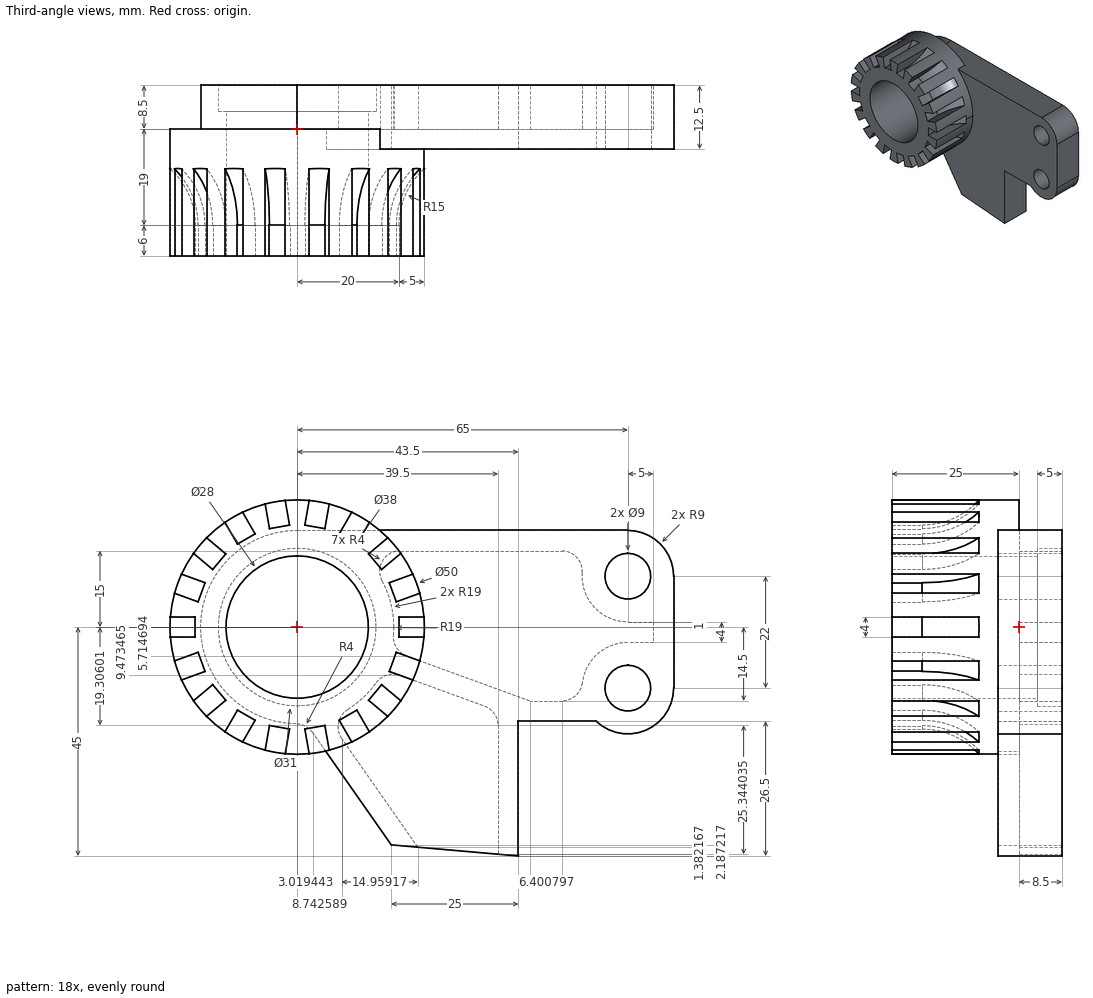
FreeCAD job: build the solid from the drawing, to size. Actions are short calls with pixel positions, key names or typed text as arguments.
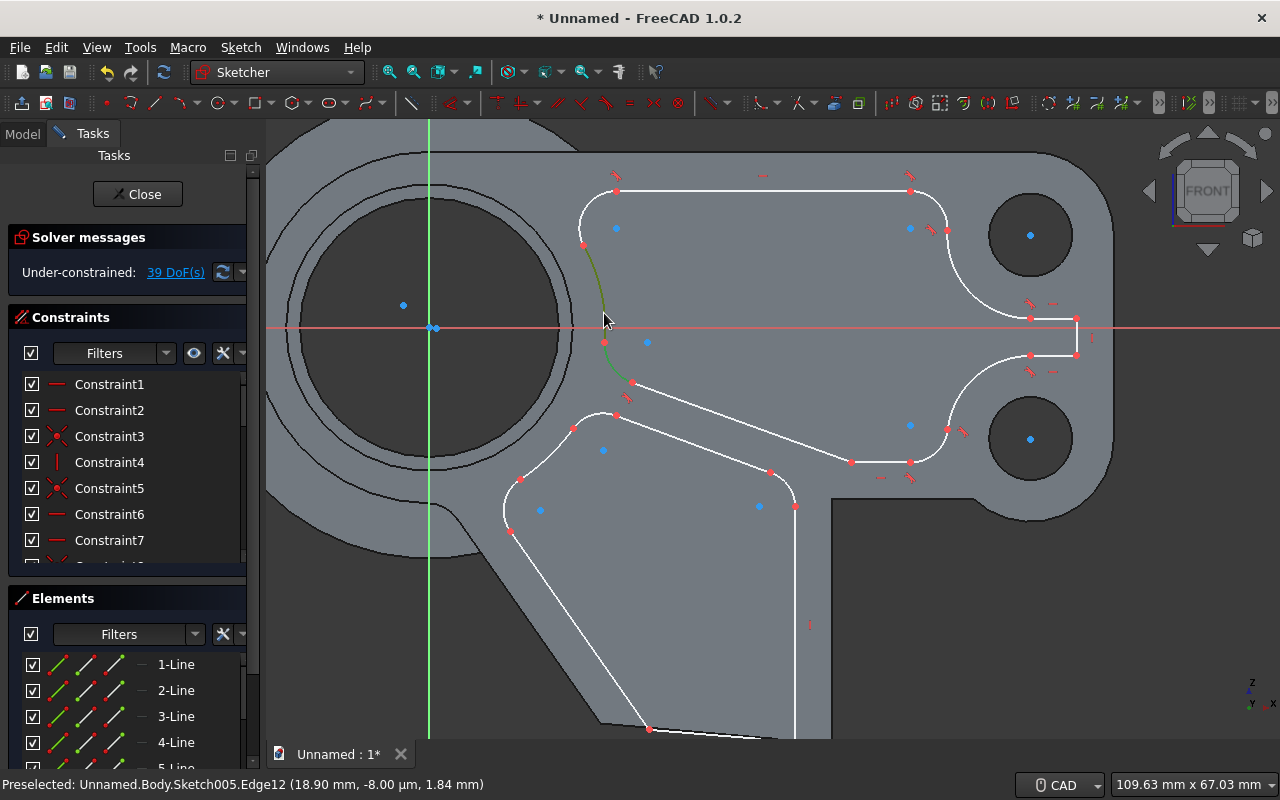
click(606, 104)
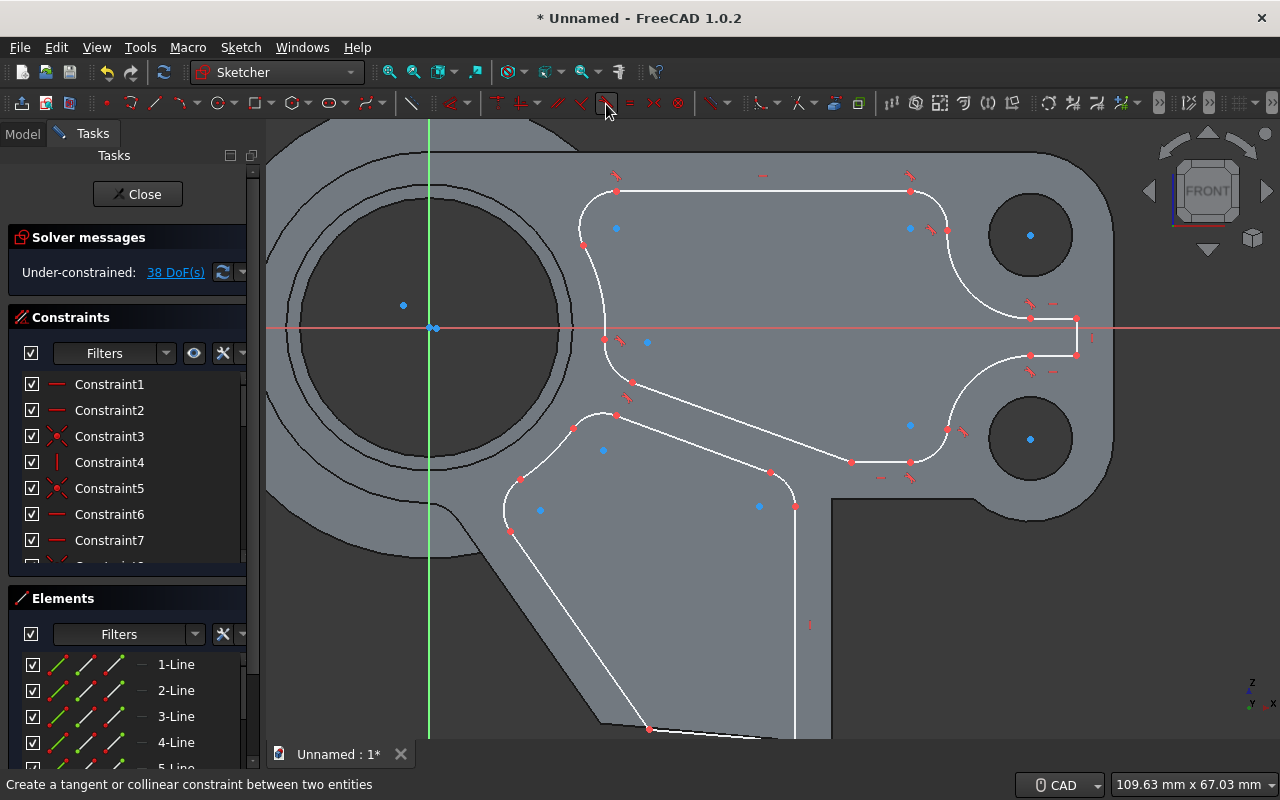
click(604, 310)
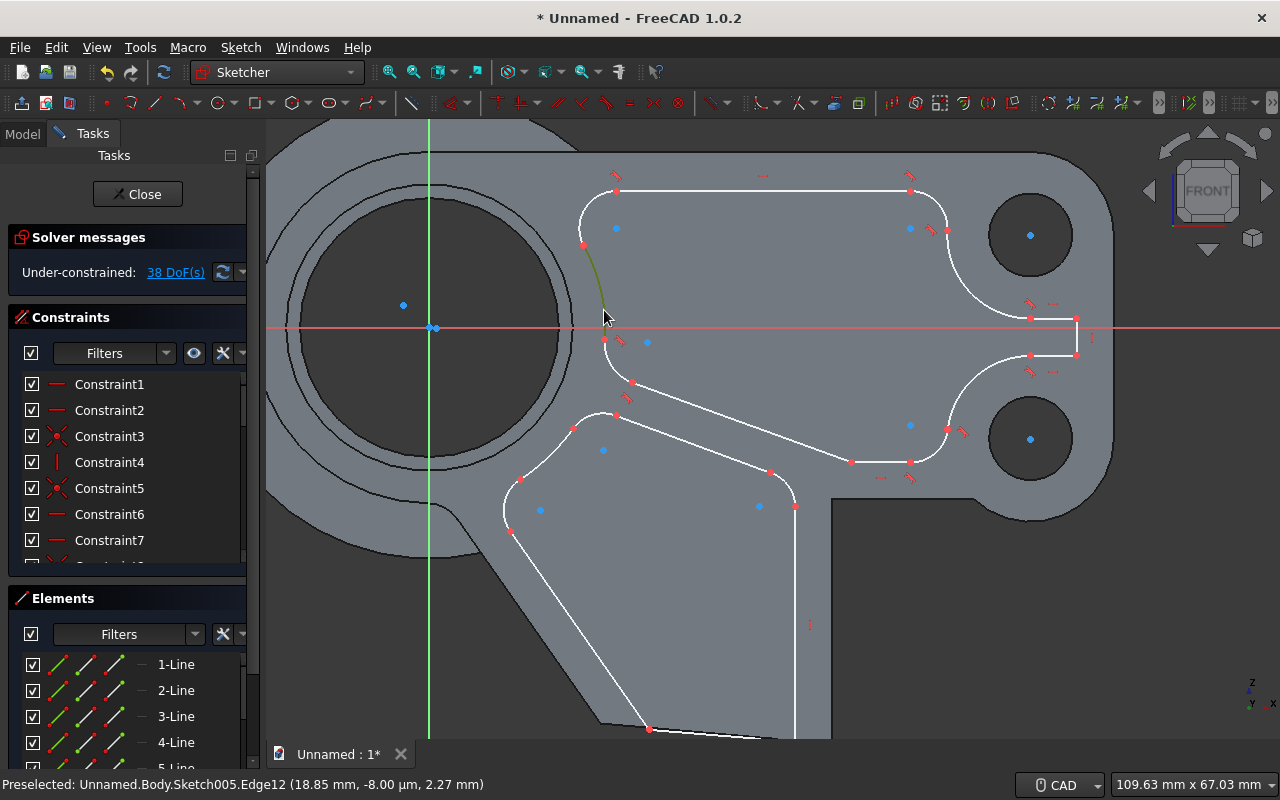
click(595, 198)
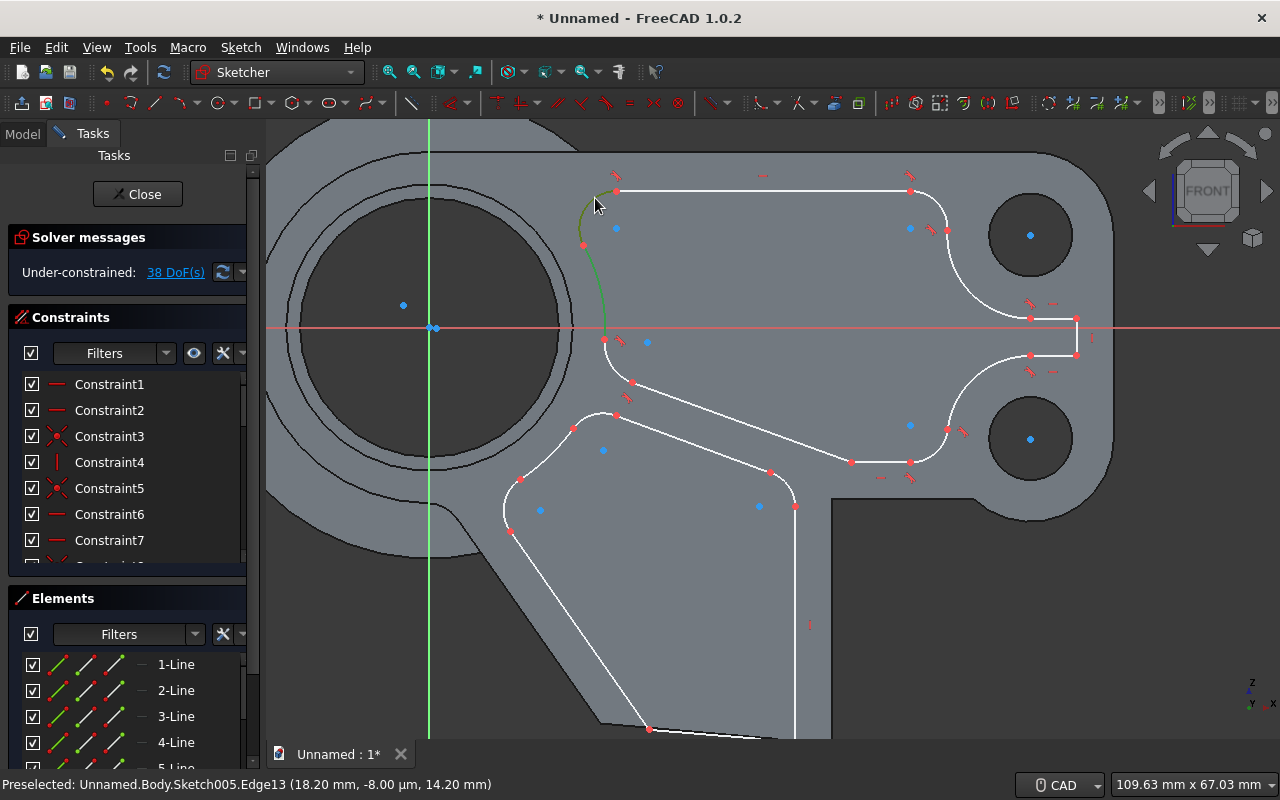
click(606, 104)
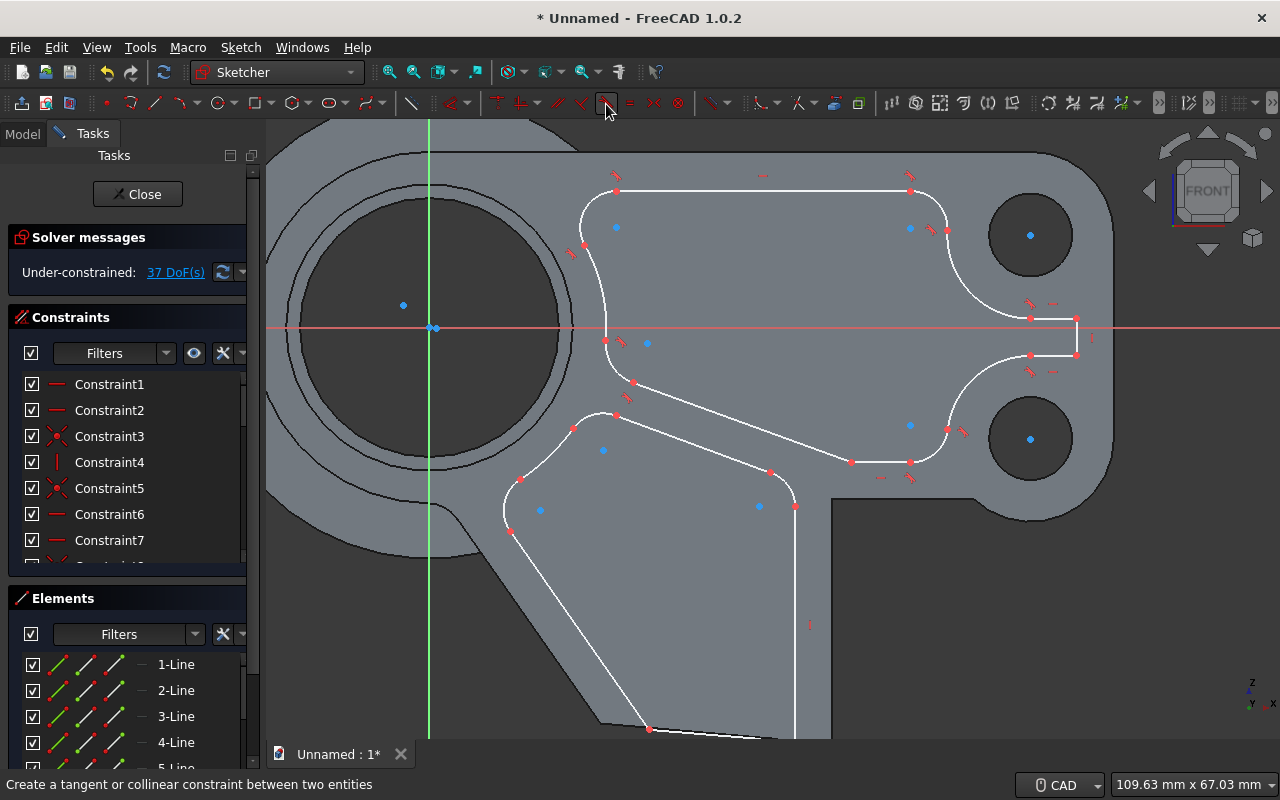
click(662, 433)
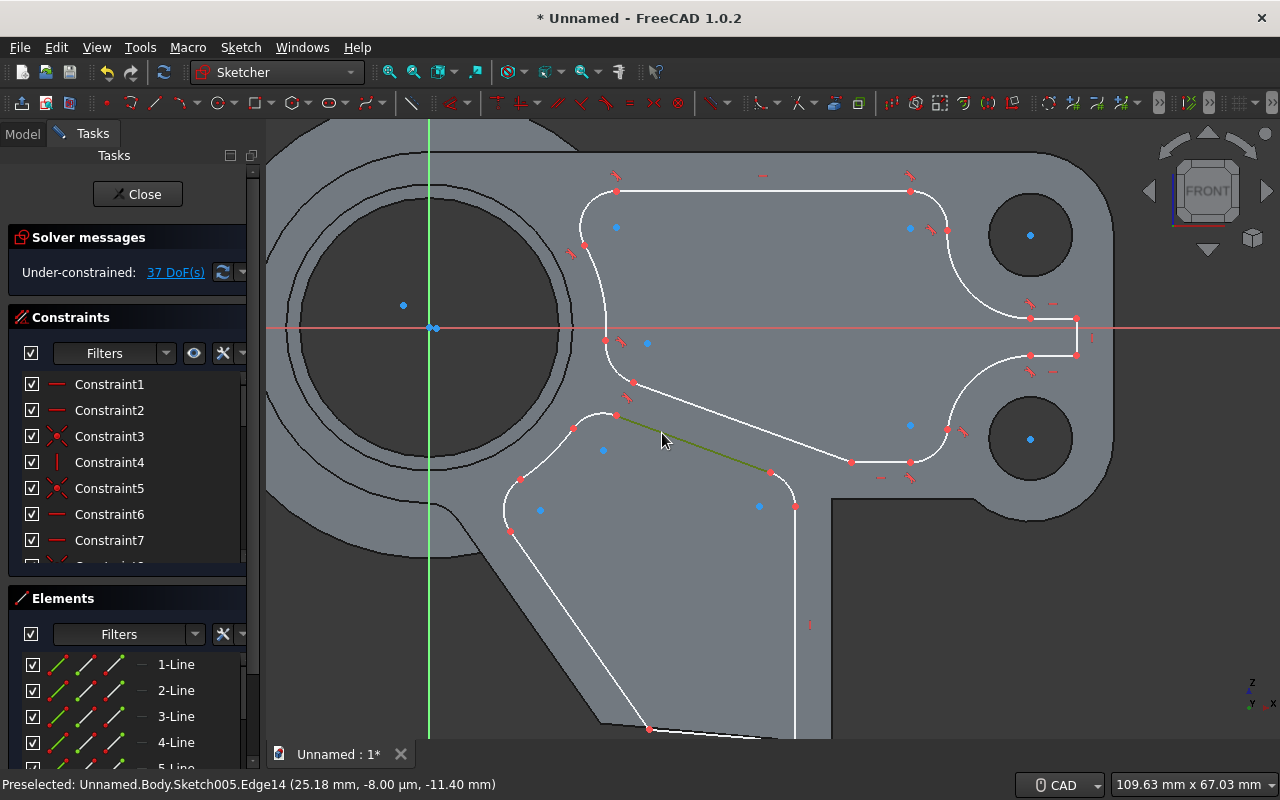
click(793, 494)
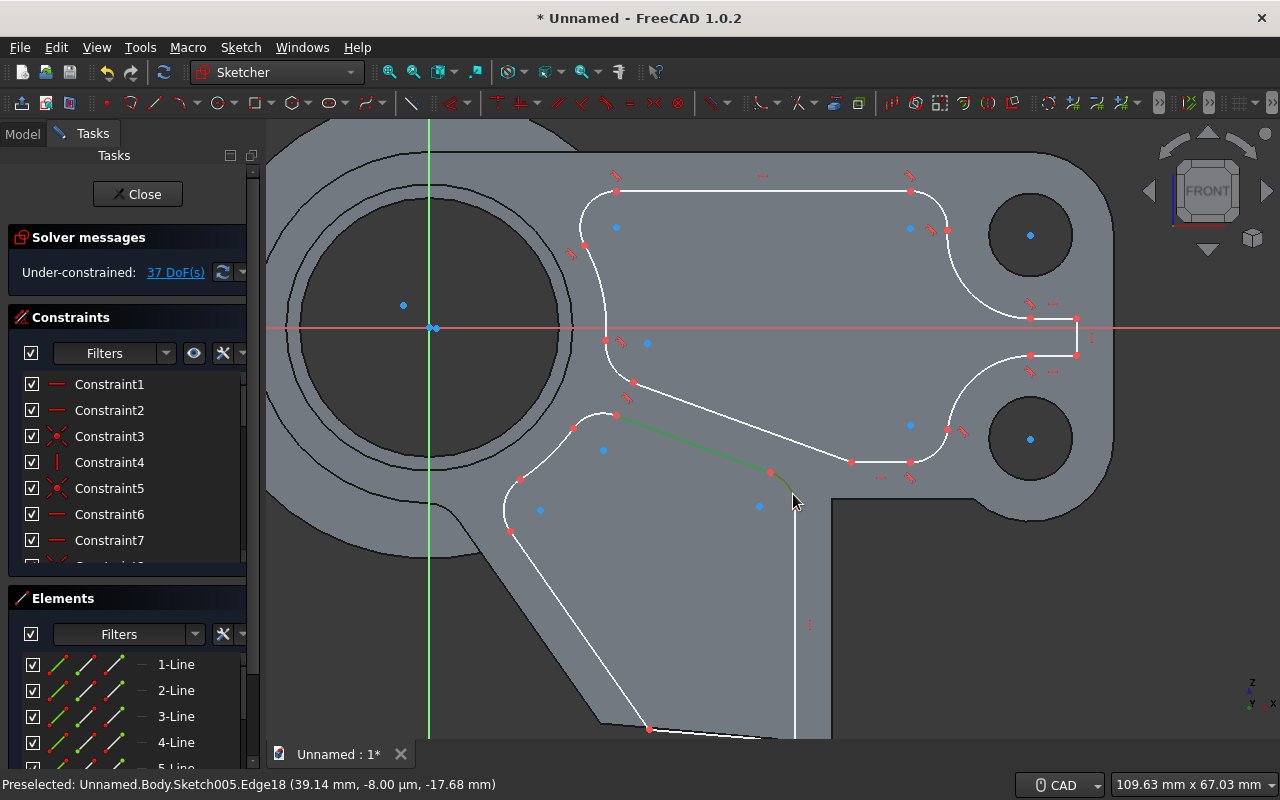
click(606, 104)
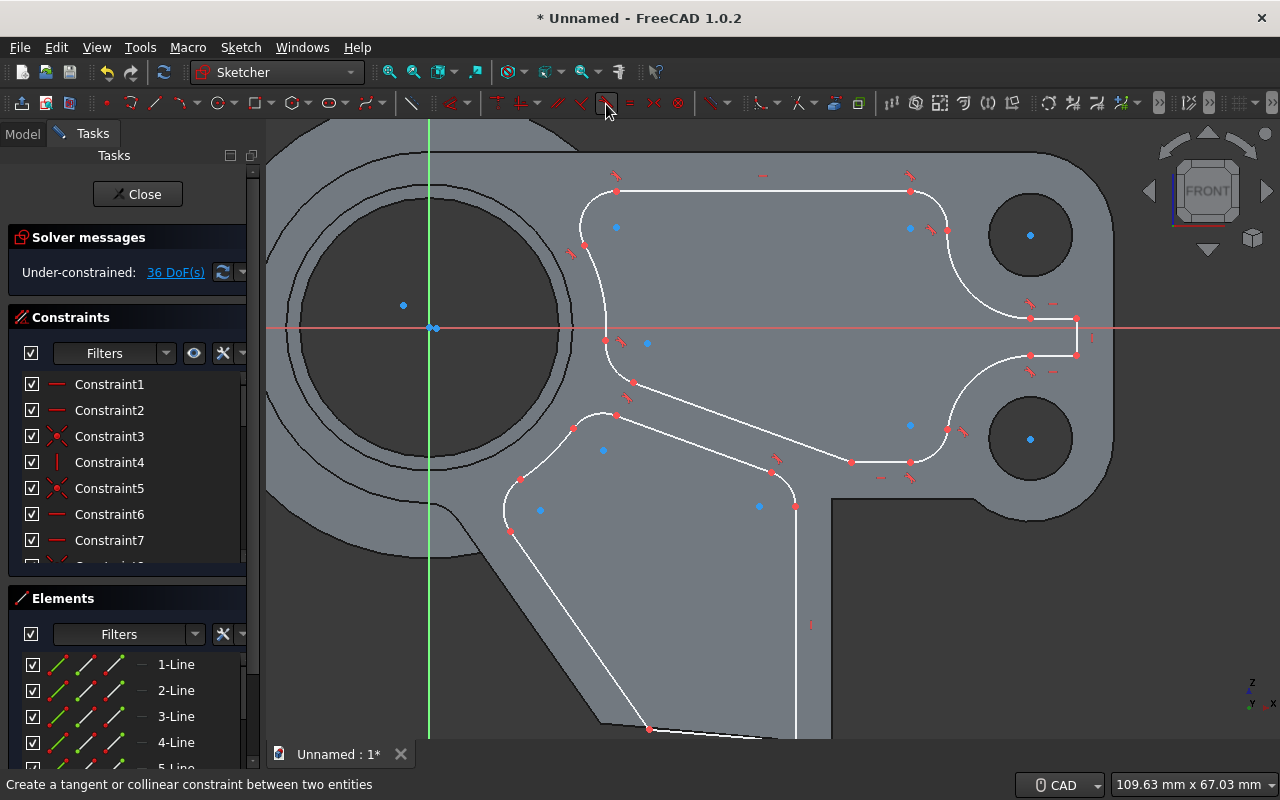
click(663, 433)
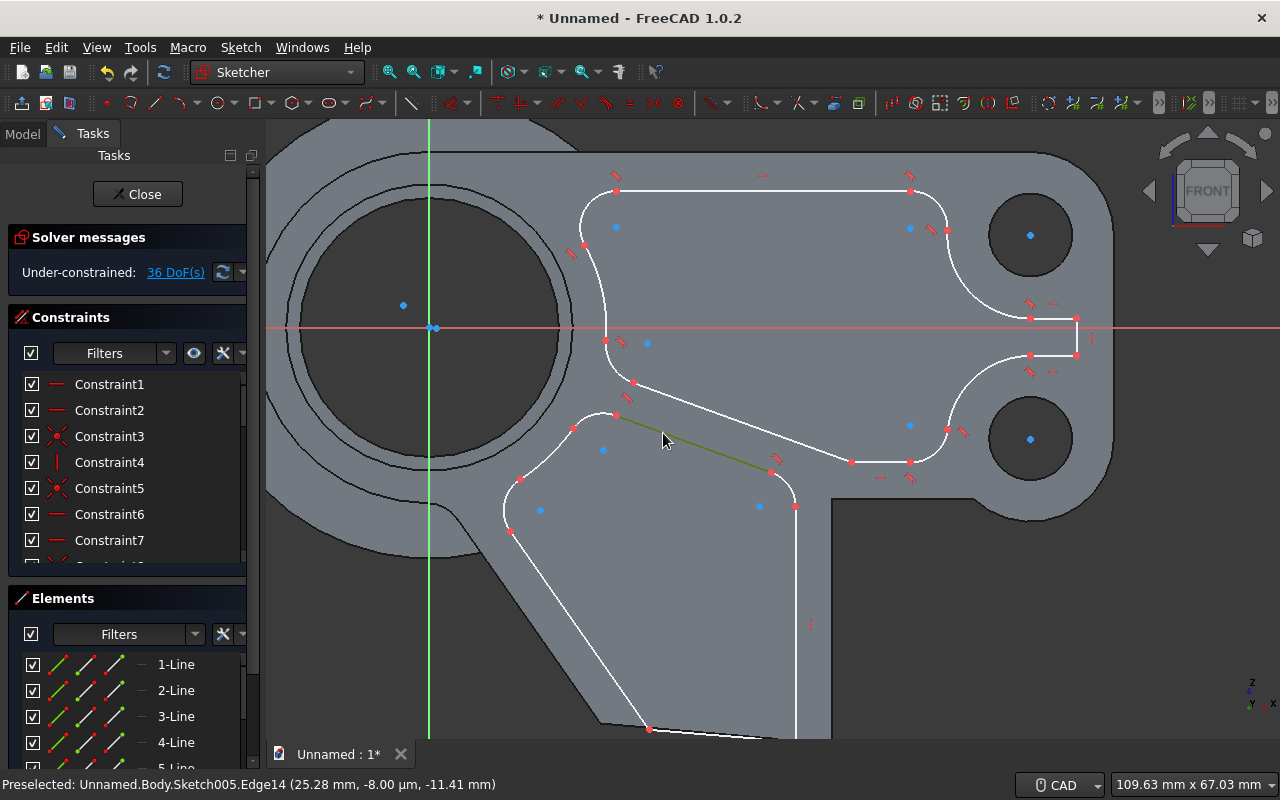
click(602, 413)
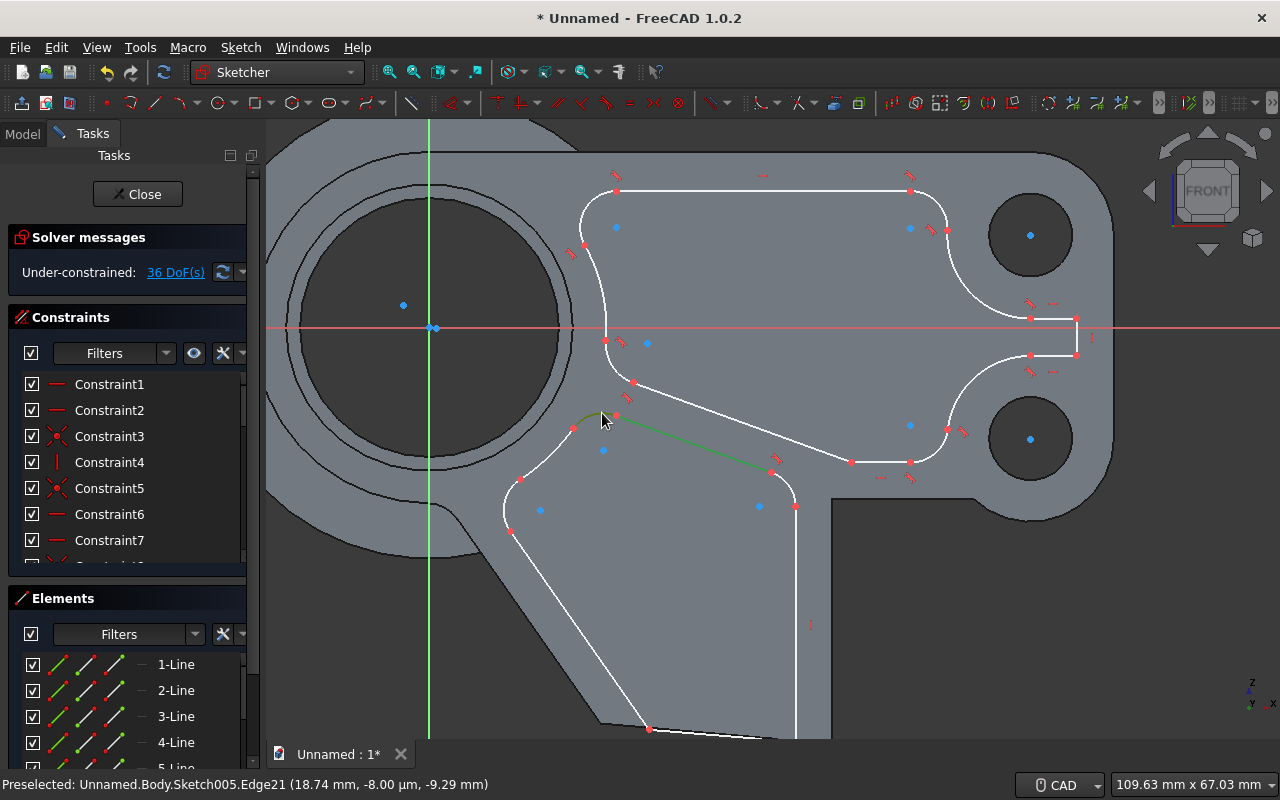
click(606, 104)